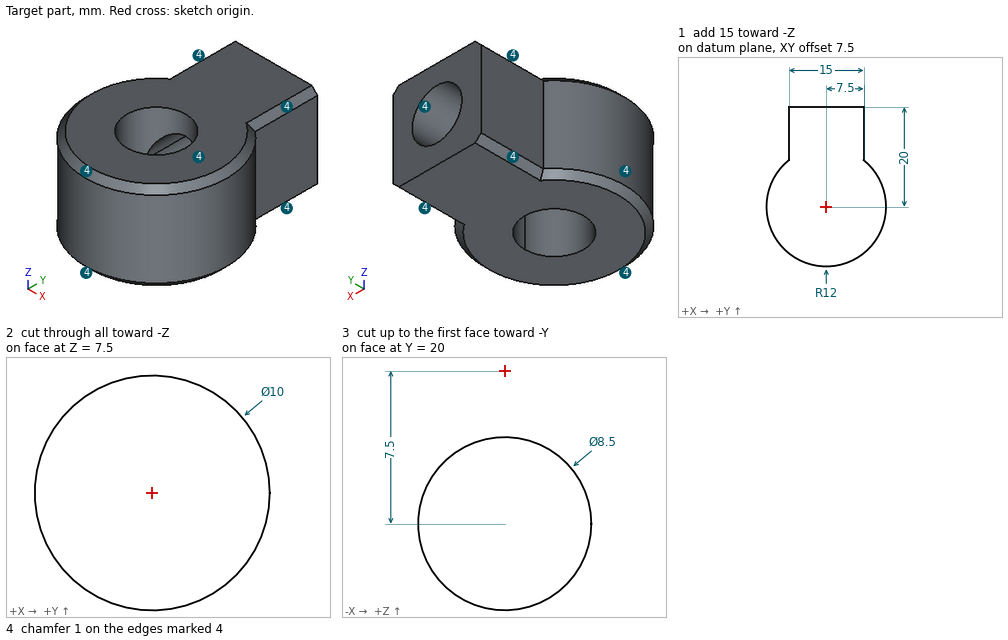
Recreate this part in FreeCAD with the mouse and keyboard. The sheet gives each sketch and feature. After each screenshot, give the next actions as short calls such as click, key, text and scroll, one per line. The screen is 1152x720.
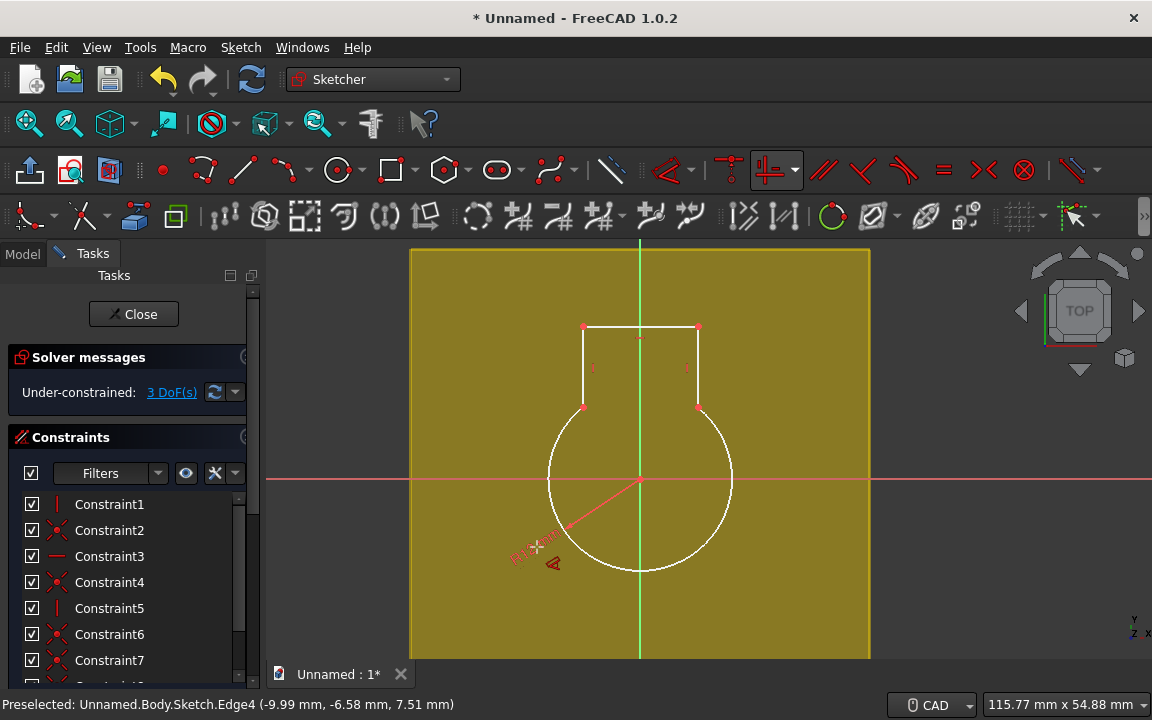
click(664, 327)
click(614, 293)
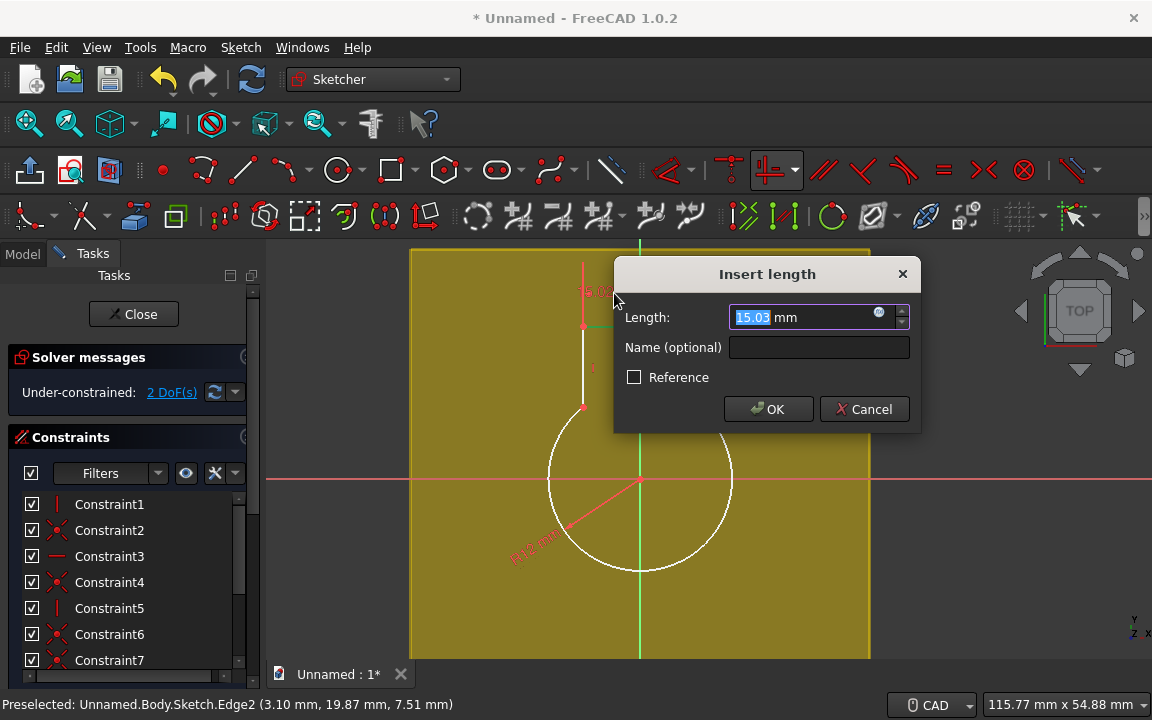
text(15)
key(Return)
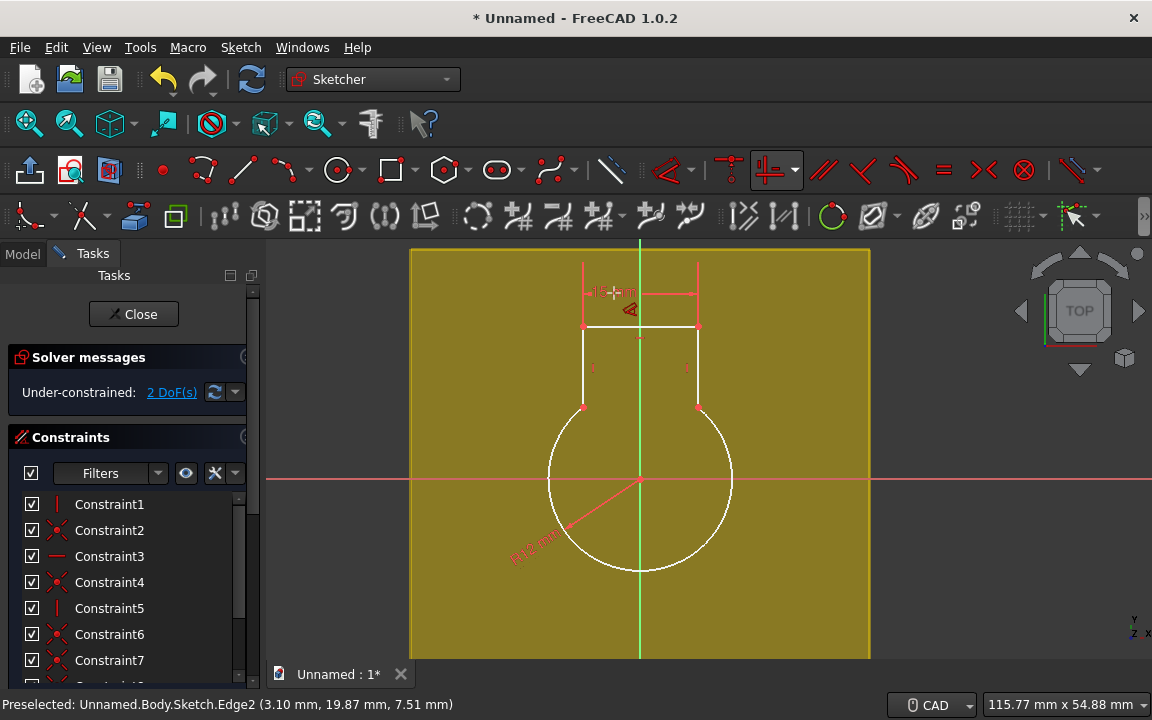
click(698, 327)
click(732, 403)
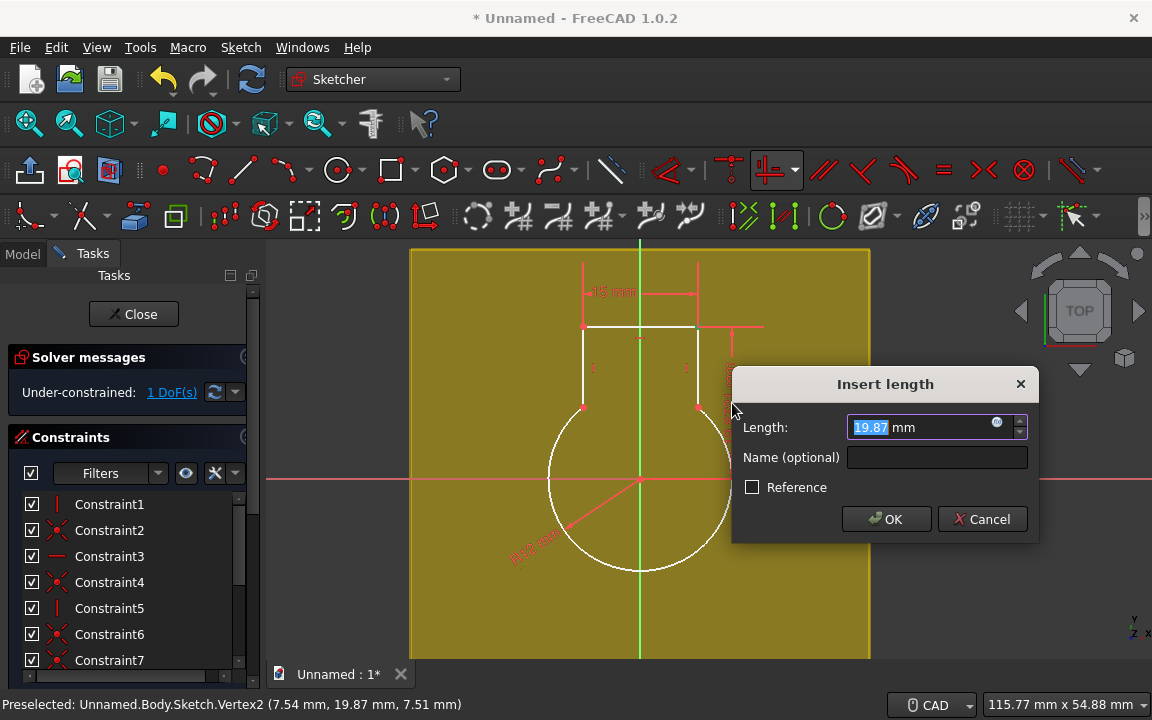
text(20)
key(Return)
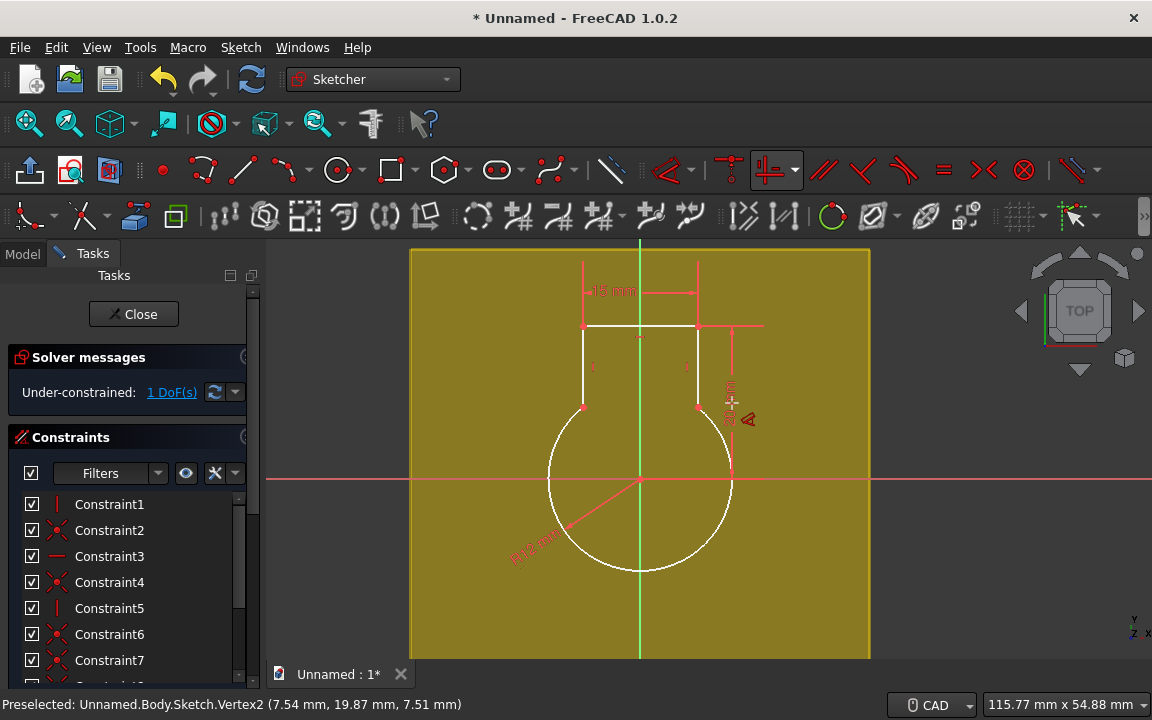
click(698, 408)
click(669, 374)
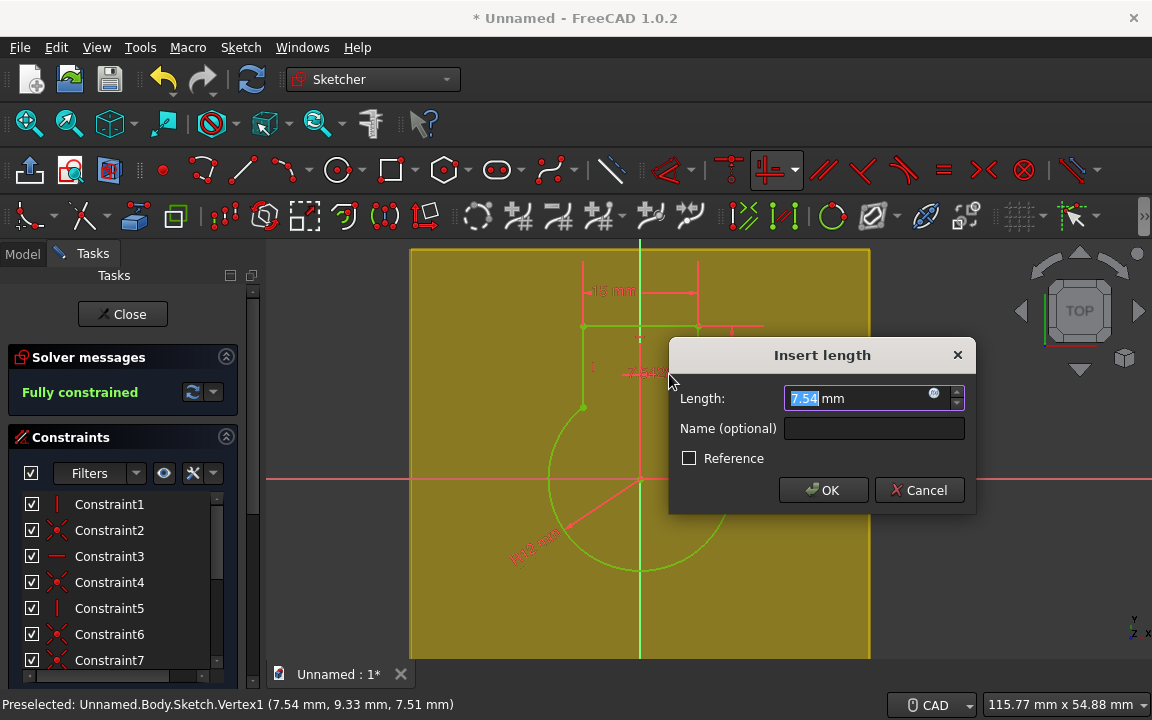
text(7.5)
key(Return)
key(Escape)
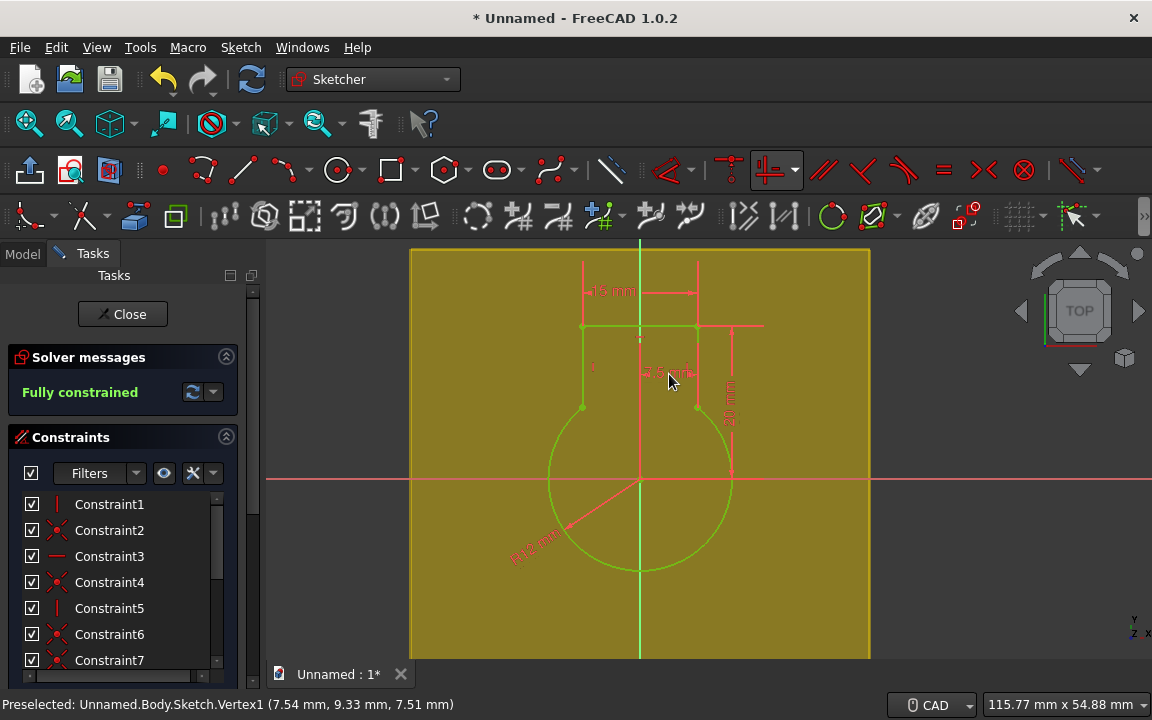
click(123, 314)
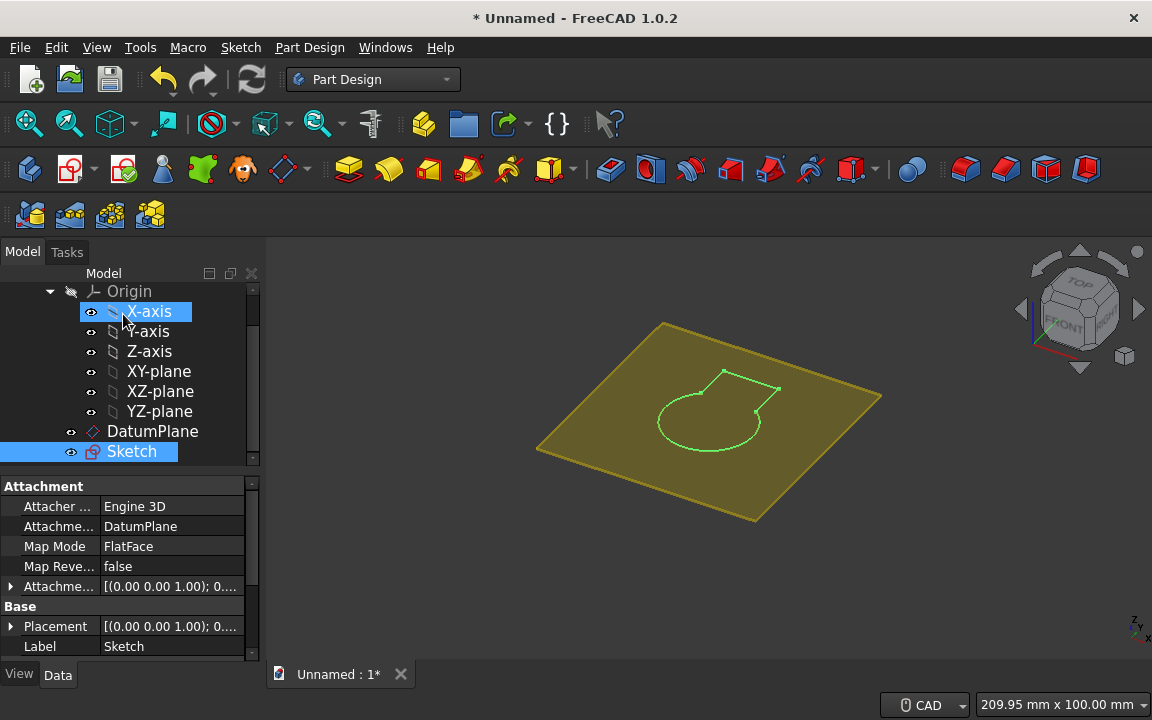
click(350, 170)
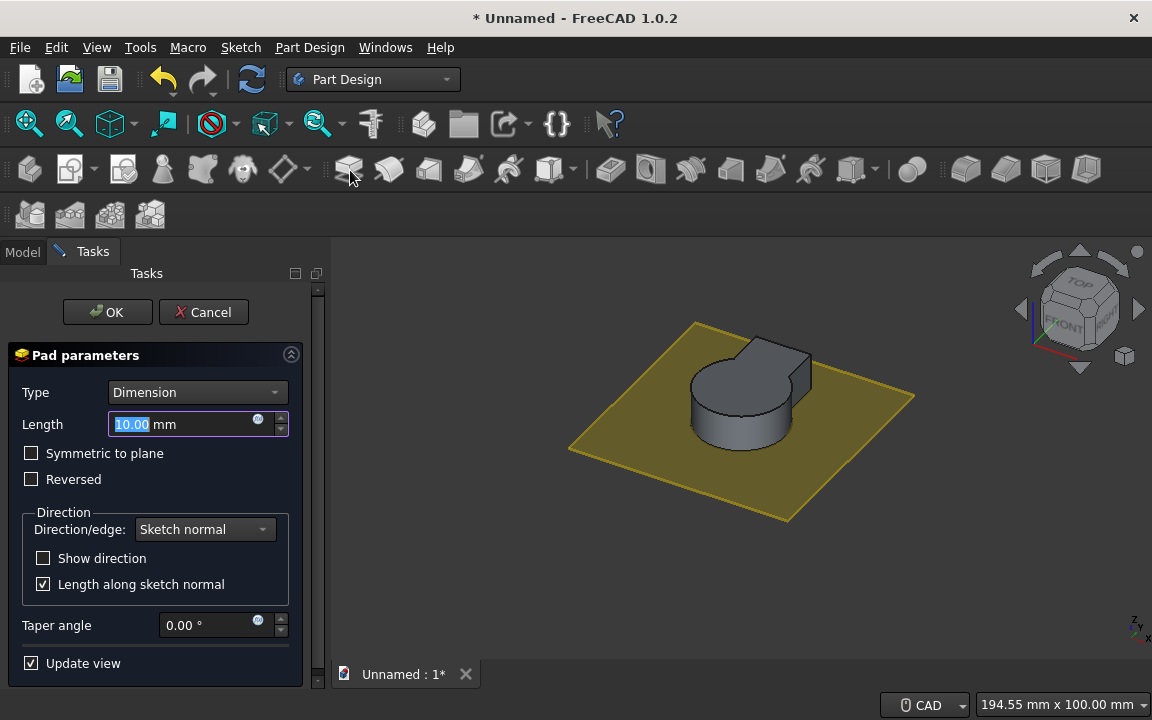
text(15)
key(Tab)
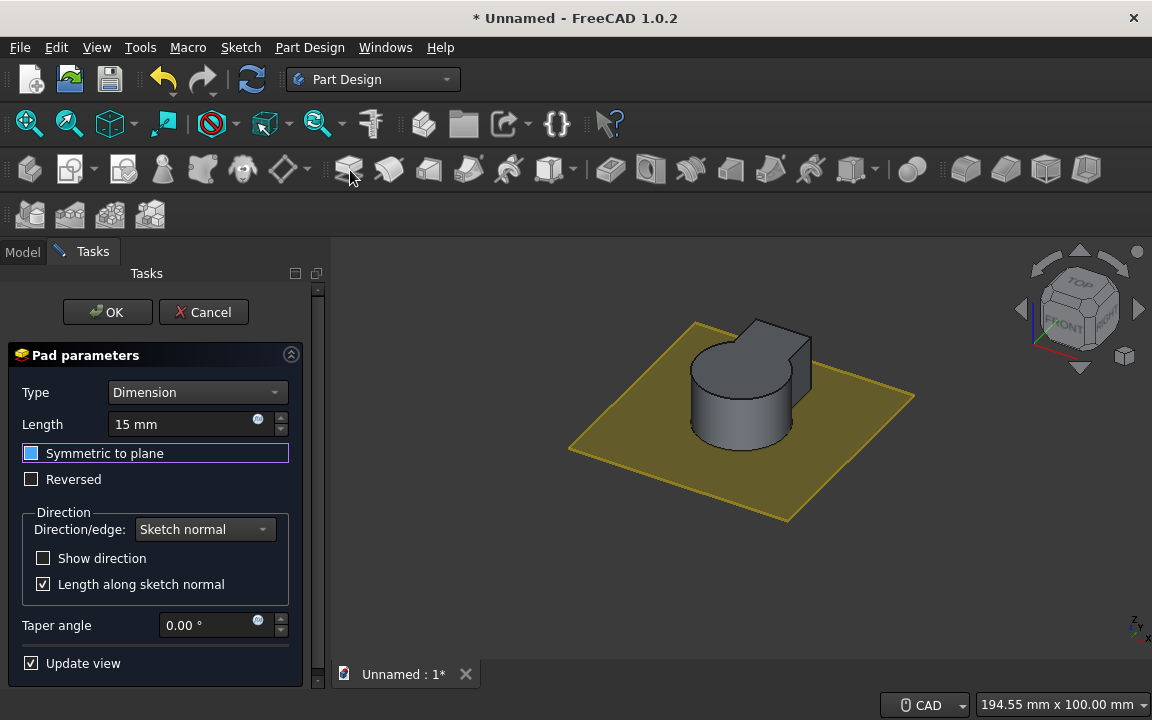
click(30, 479)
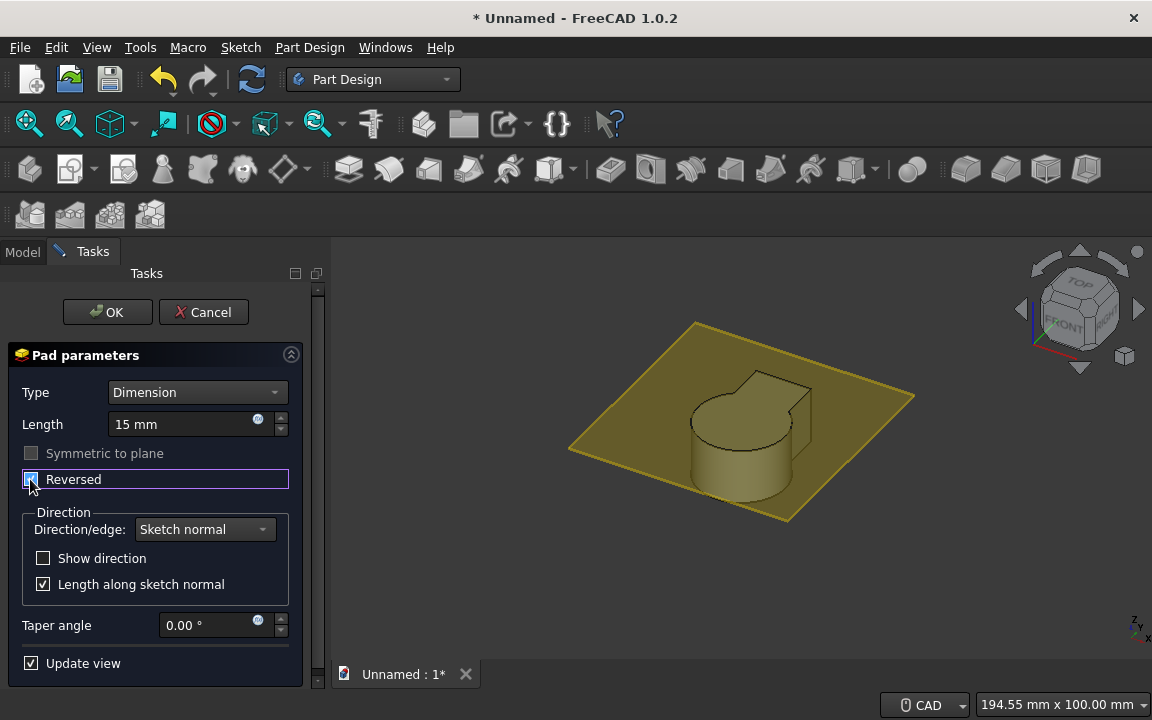
click(108, 312)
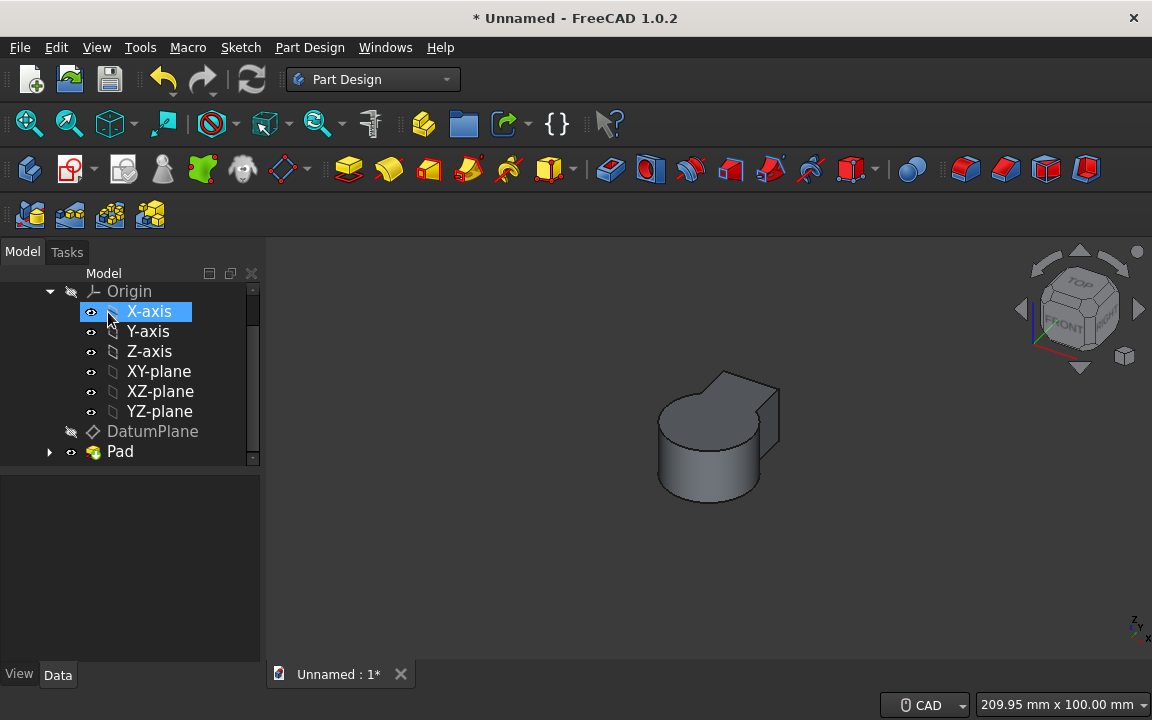
click(30, 124)